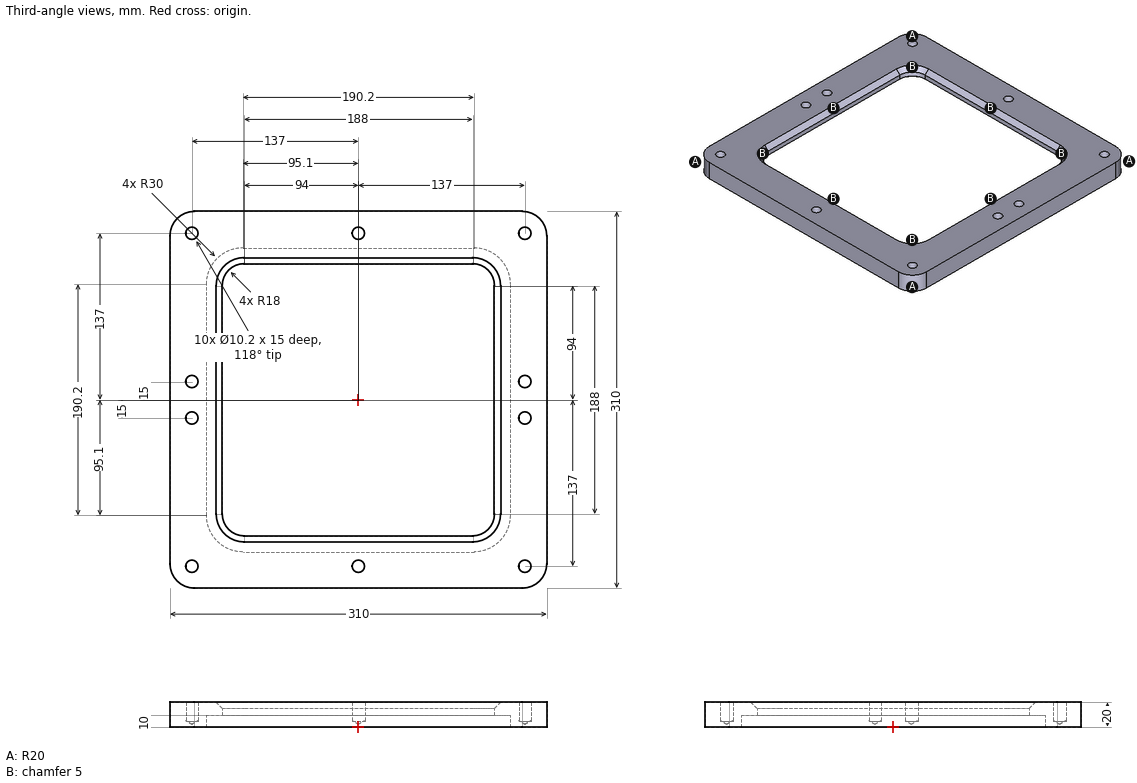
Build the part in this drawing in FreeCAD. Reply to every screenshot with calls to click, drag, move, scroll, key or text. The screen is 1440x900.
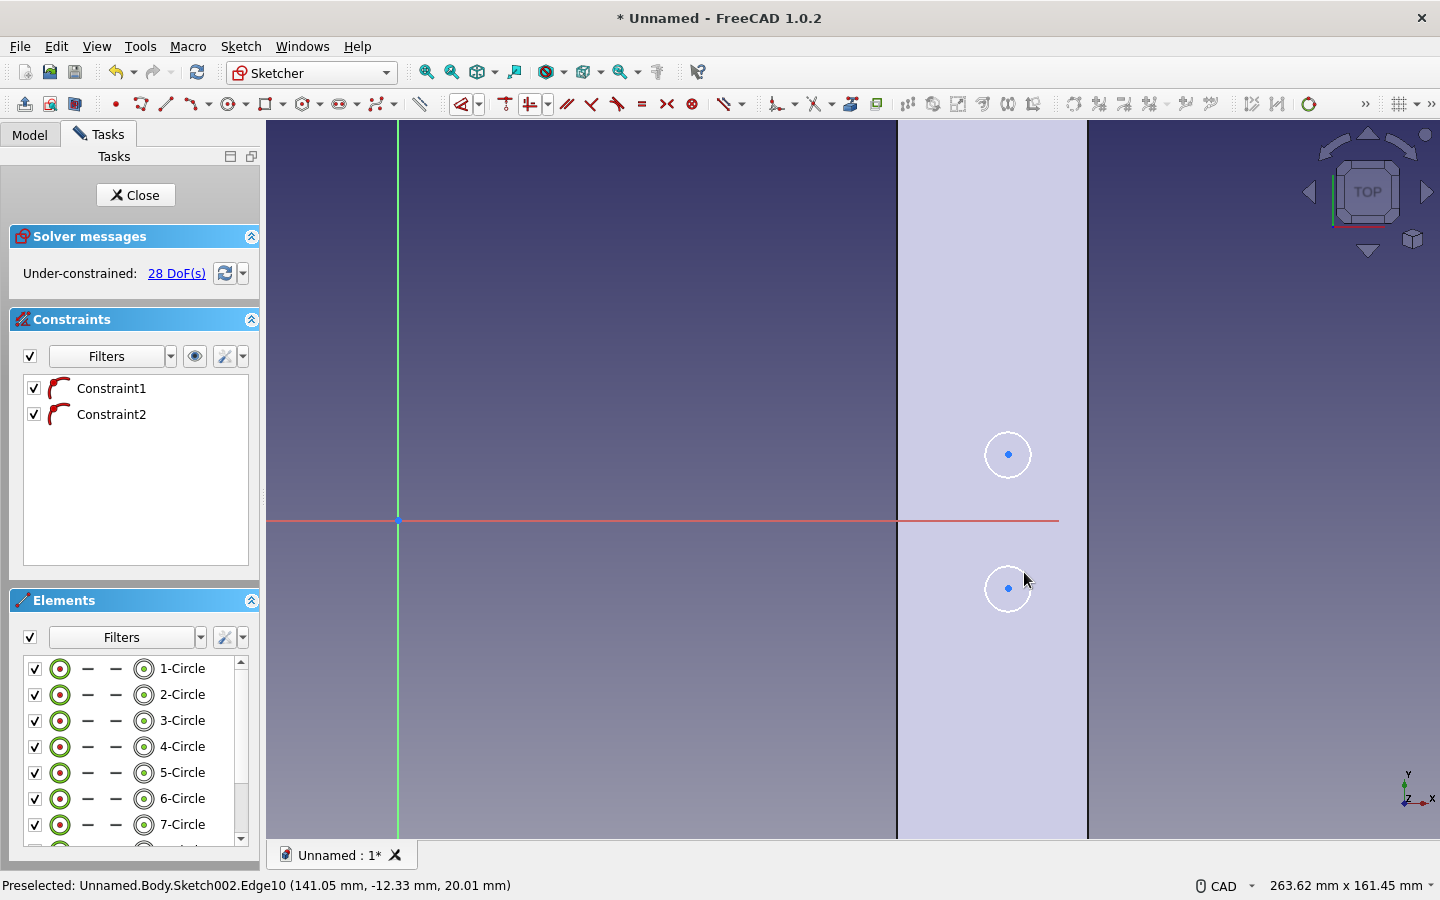
scroll(1009, 455, down, 5)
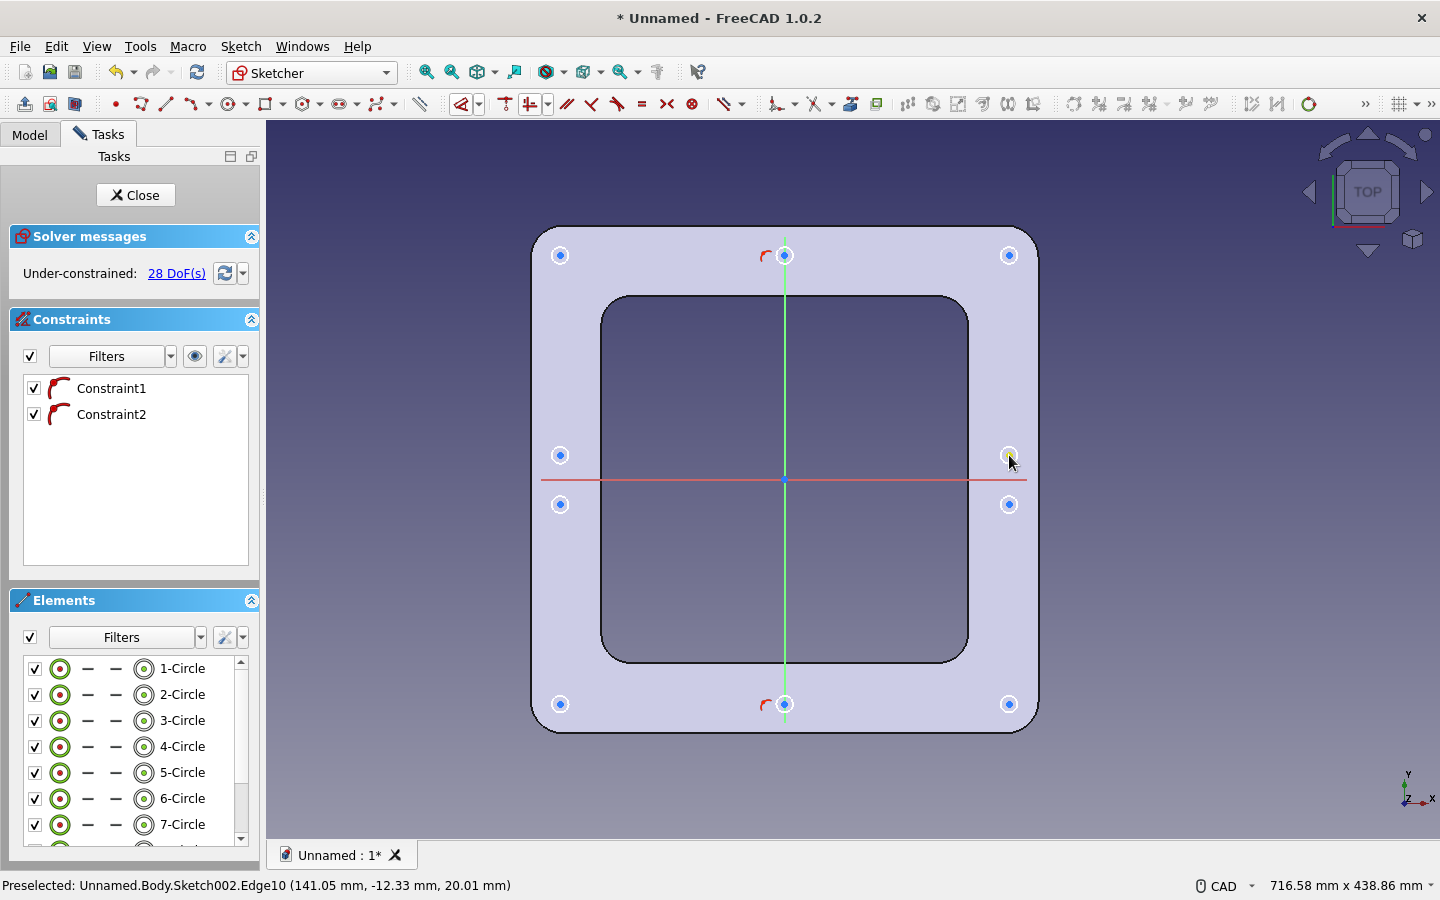
scroll(566, 250, up, 3)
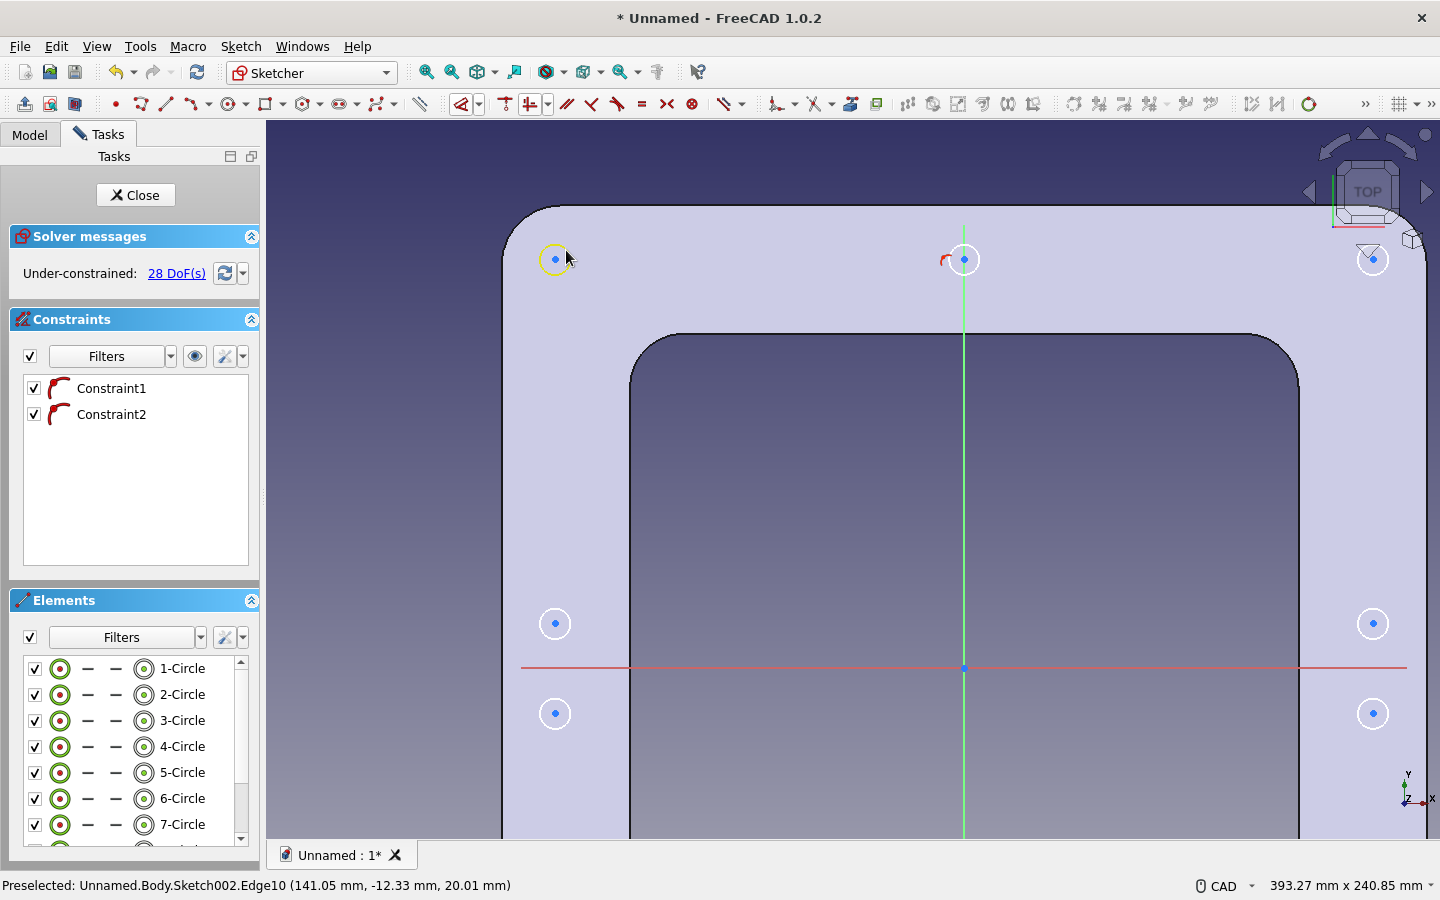
click(566, 249)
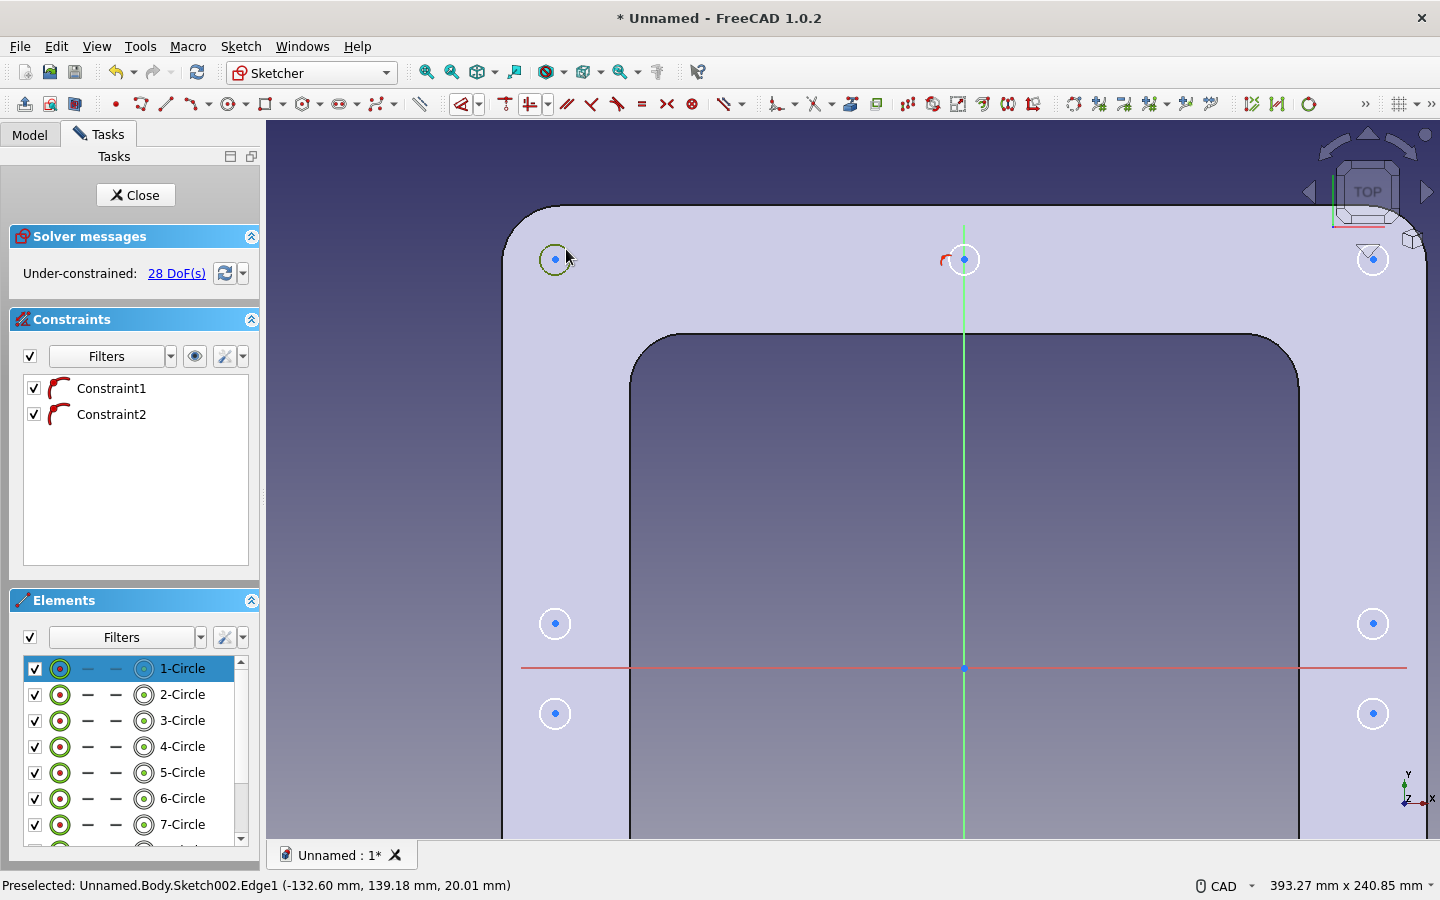
scroll(566, 250, down, 3)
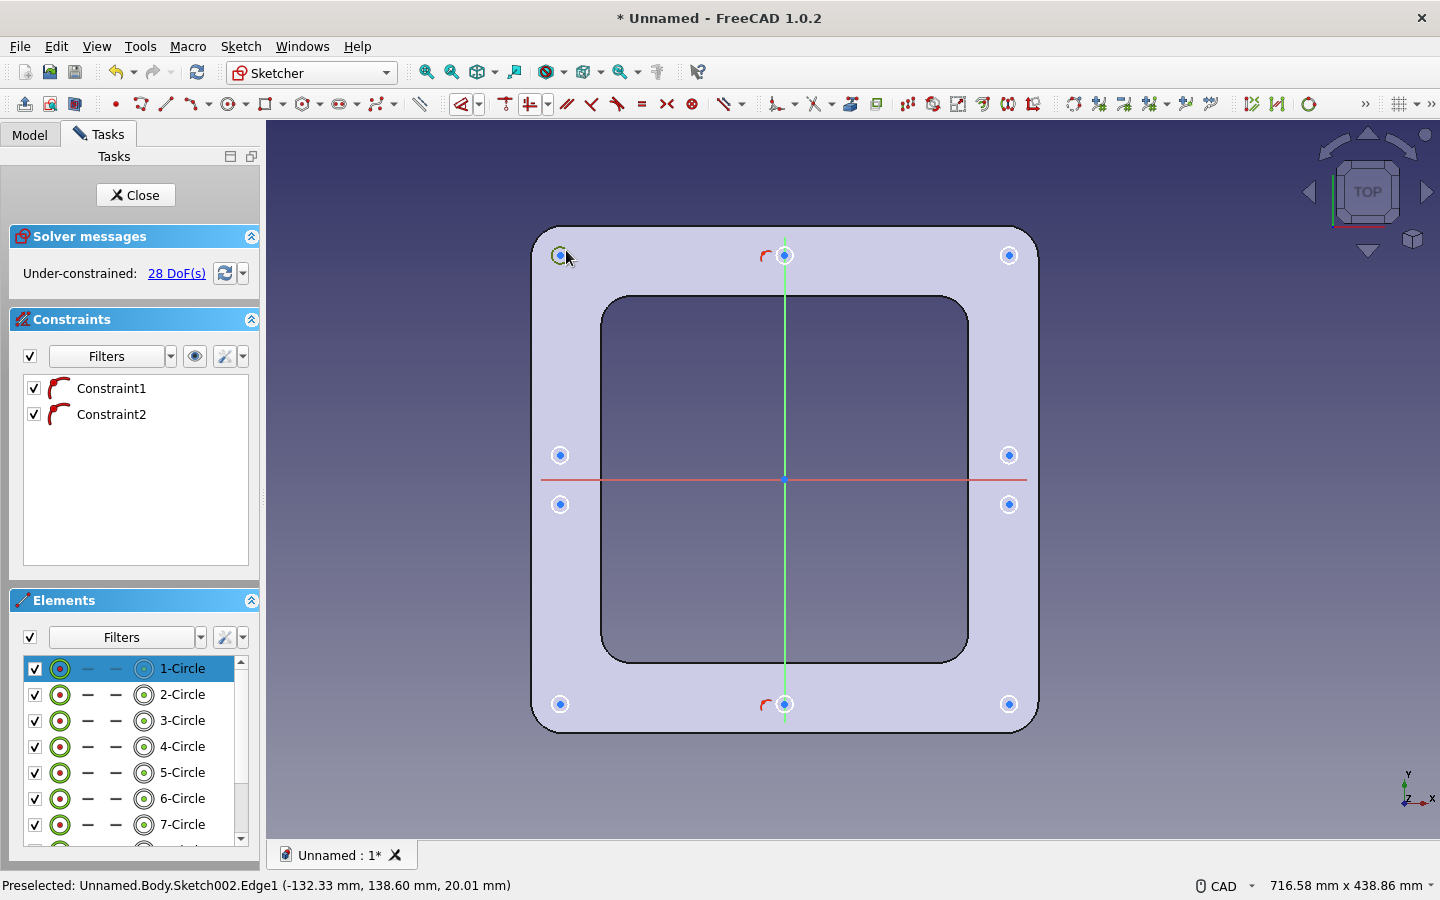
scroll(1015, 250, up, 3)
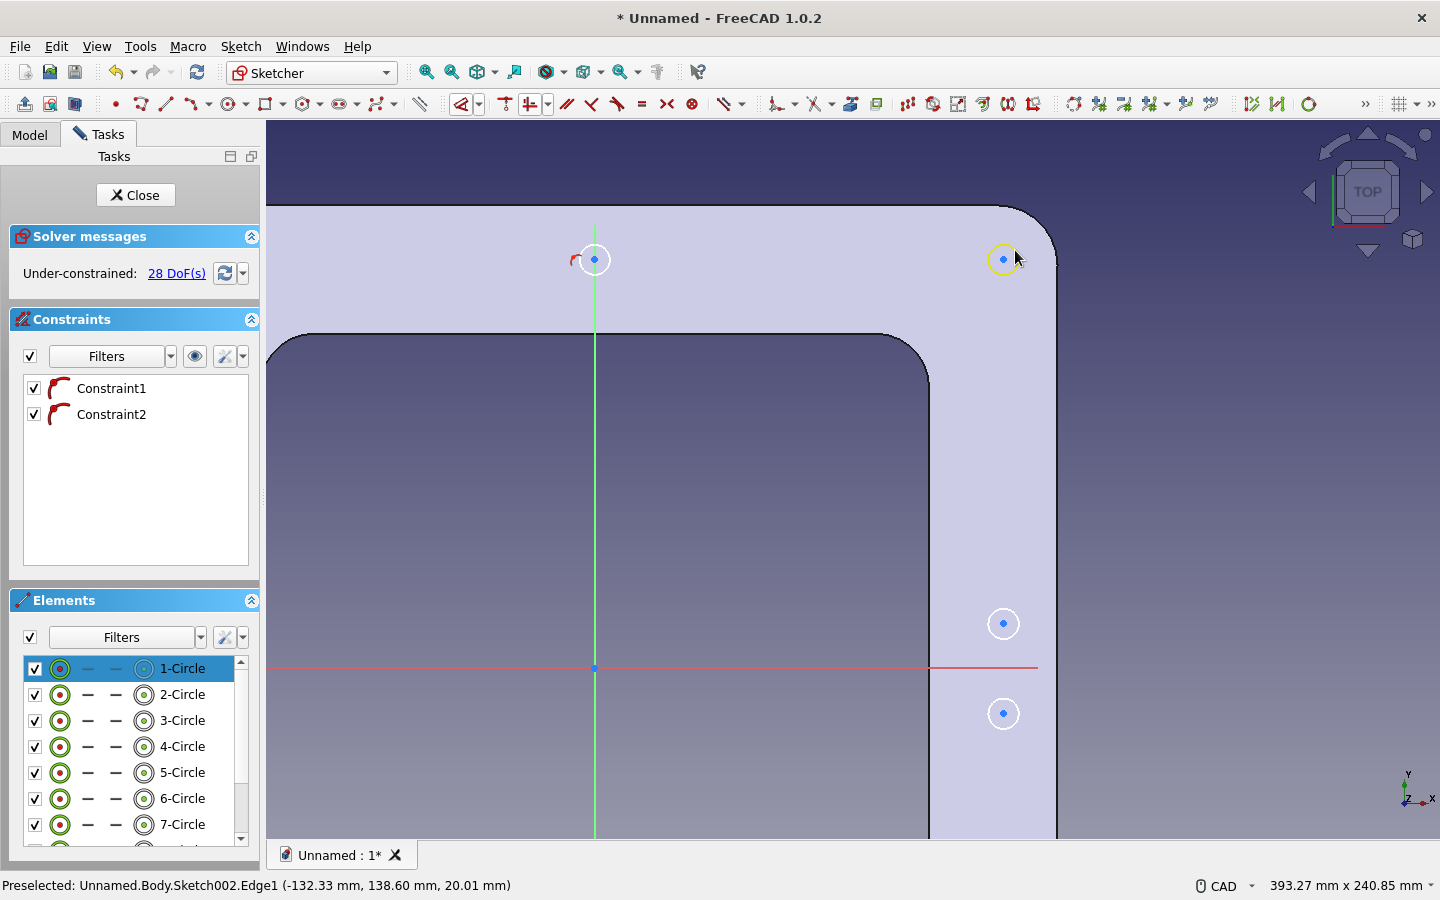
click(1014, 249)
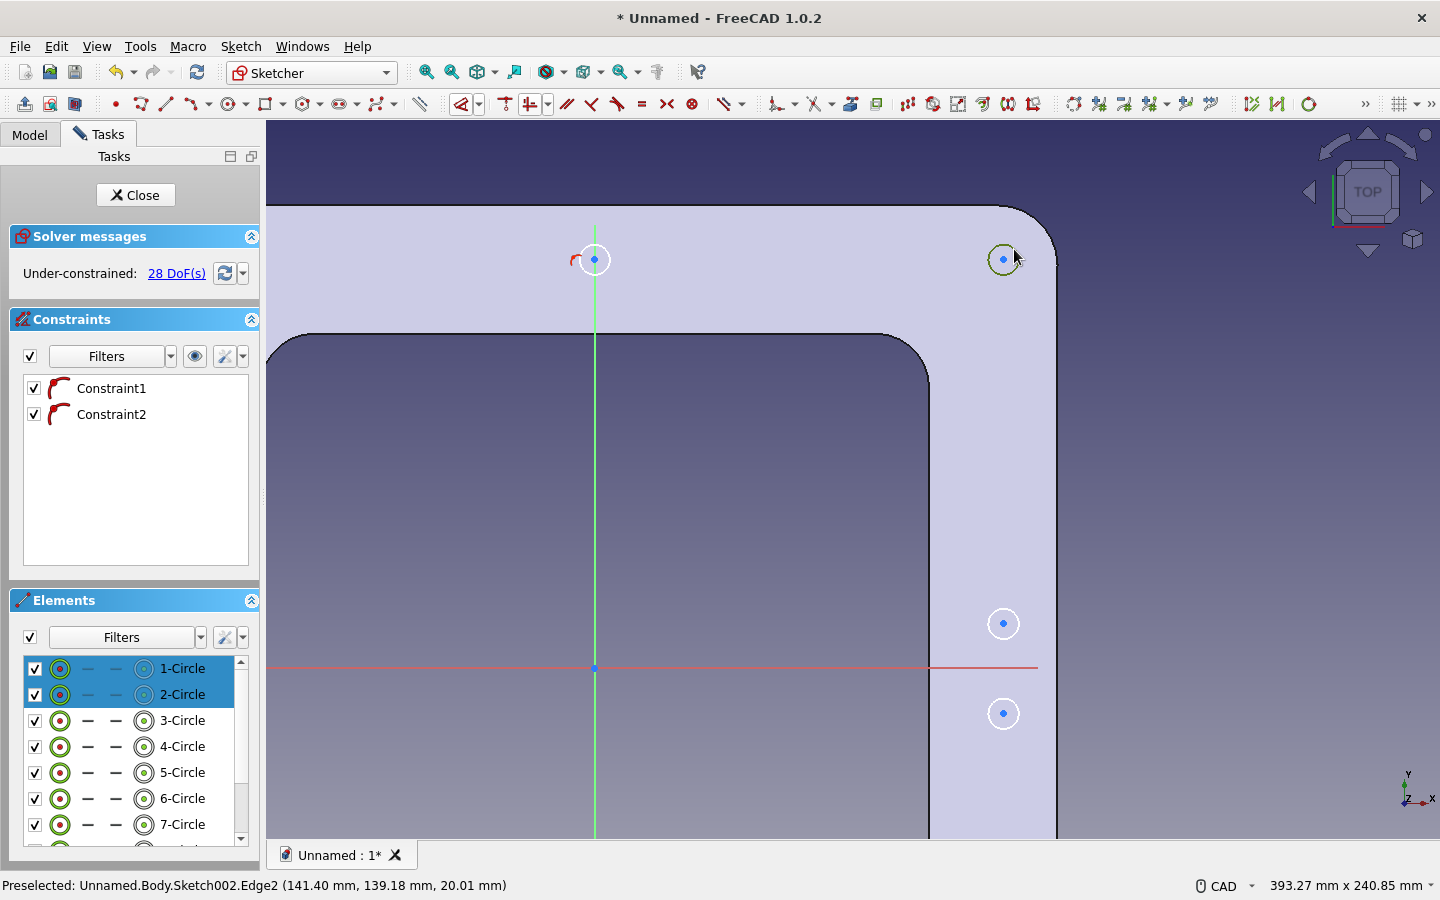
scroll(1015, 250, down, 3)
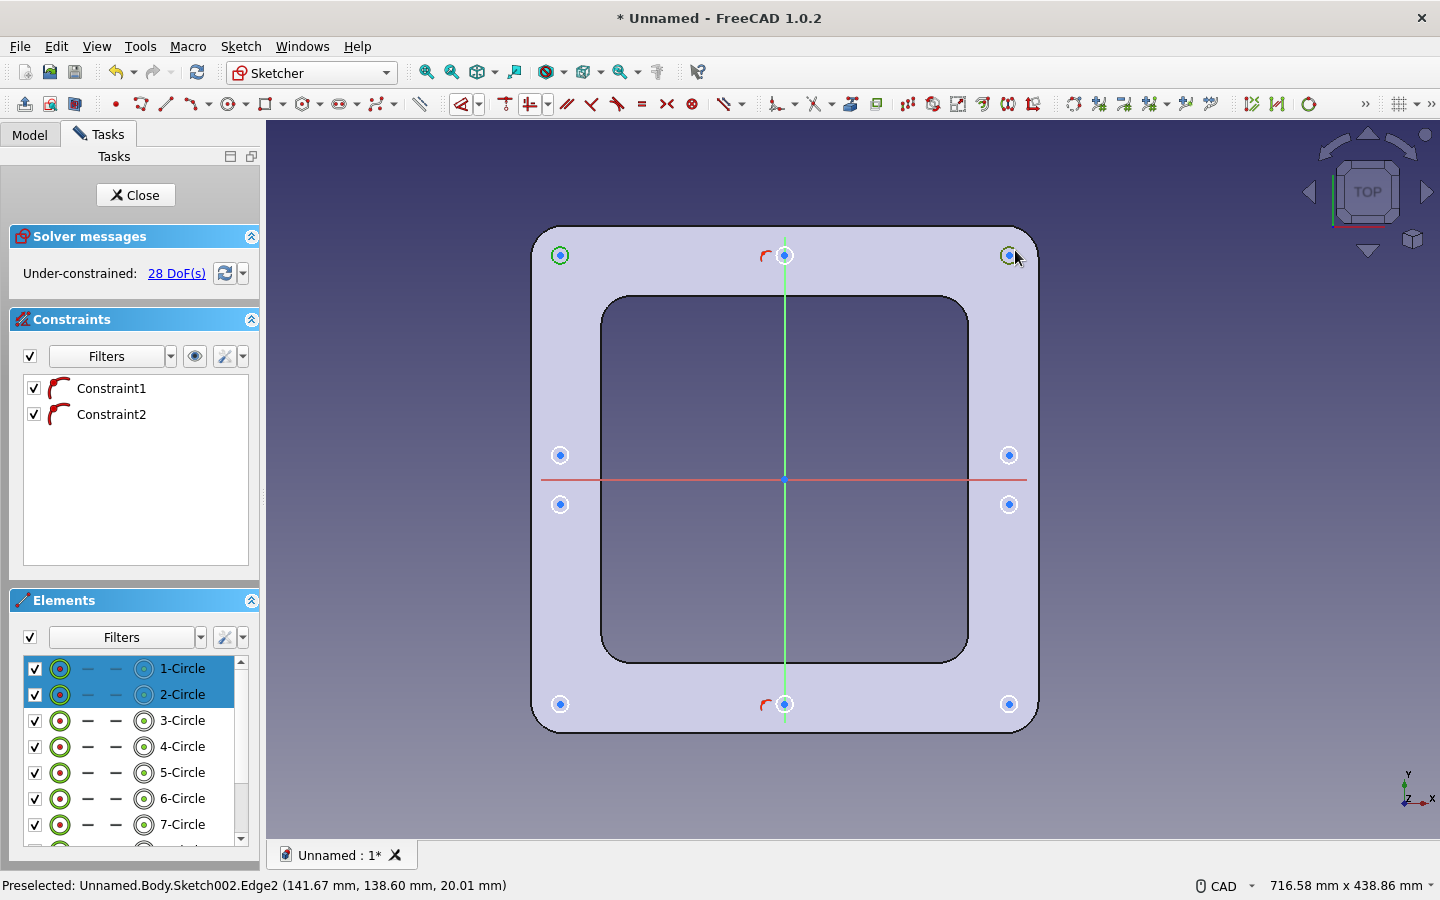
scroll(1015, 698, up, 3)